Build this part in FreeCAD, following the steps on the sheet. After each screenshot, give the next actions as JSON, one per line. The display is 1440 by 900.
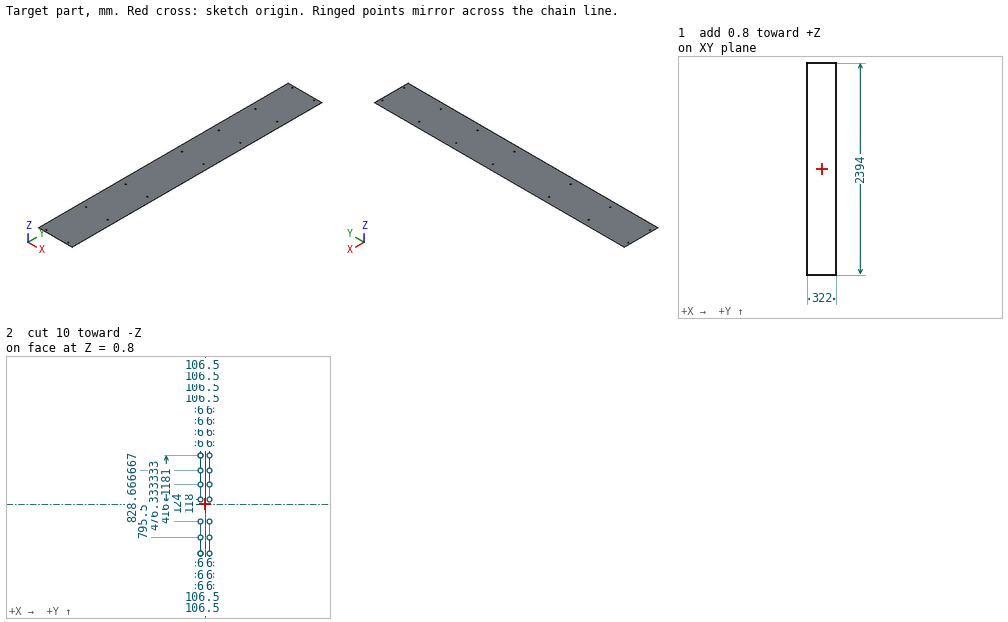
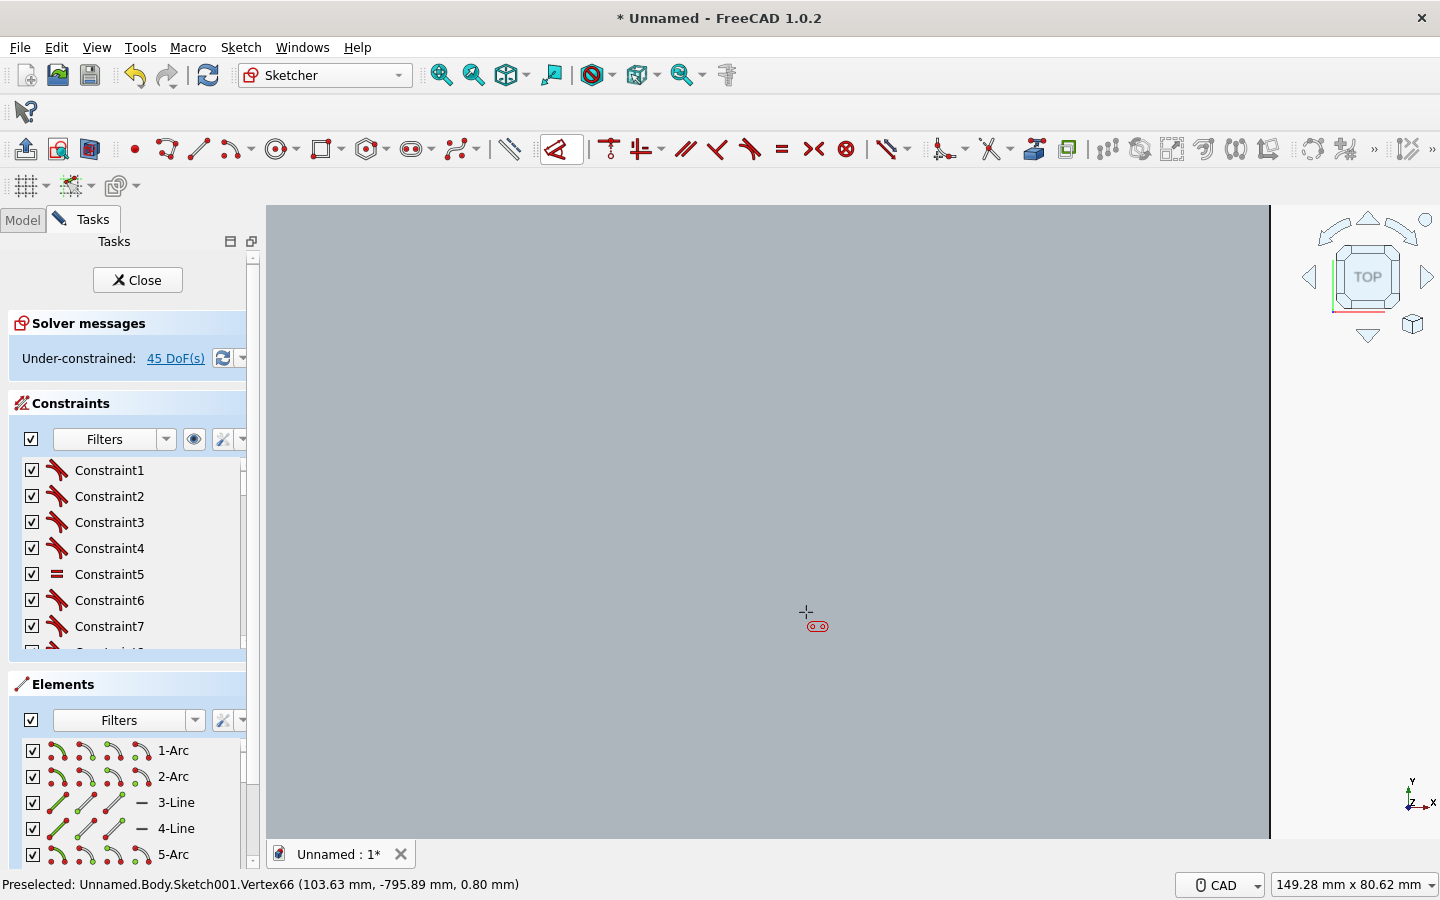
{"action": "scroll", "coordinate": [806, 612], "scroll_direction": "down", "scroll_amount": 18}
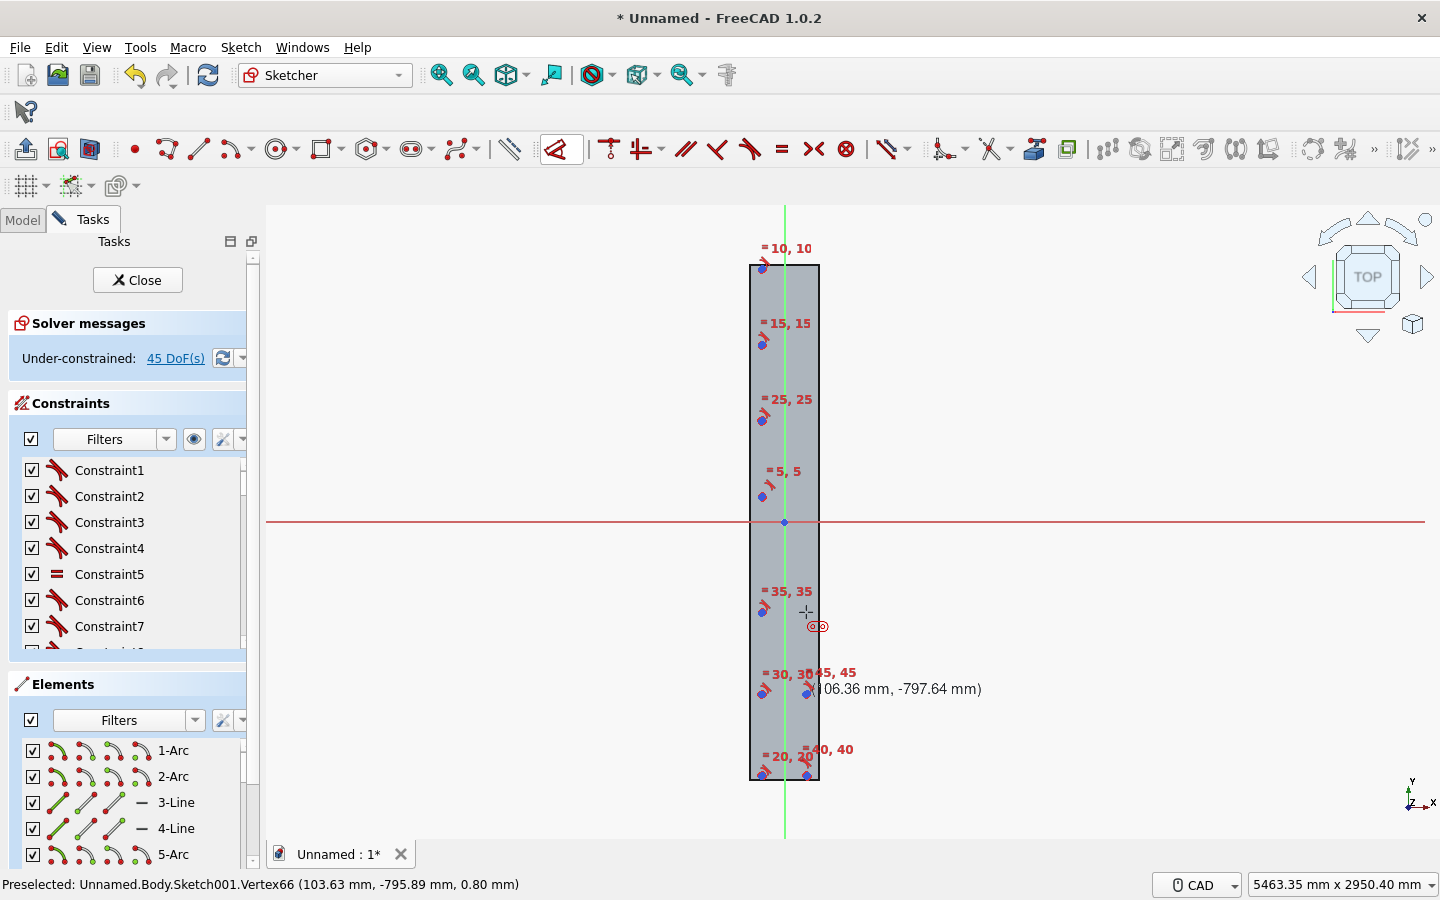
{"action": "left_click", "coordinate": [806, 612]}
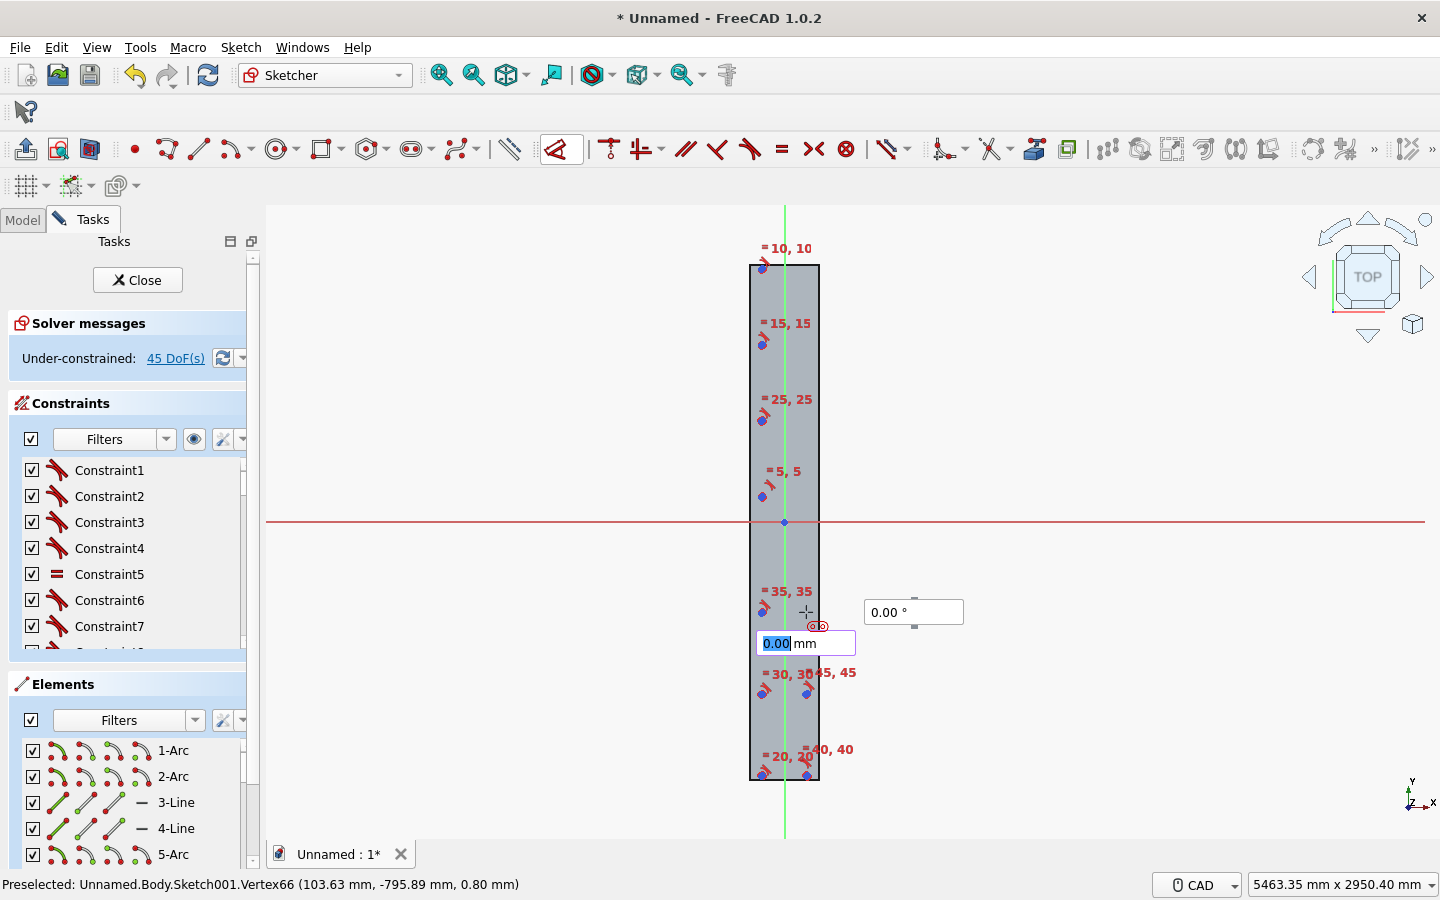
{"action": "scroll", "coordinate": [807, 612], "scroll_direction": "up", "scroll_amount": 13}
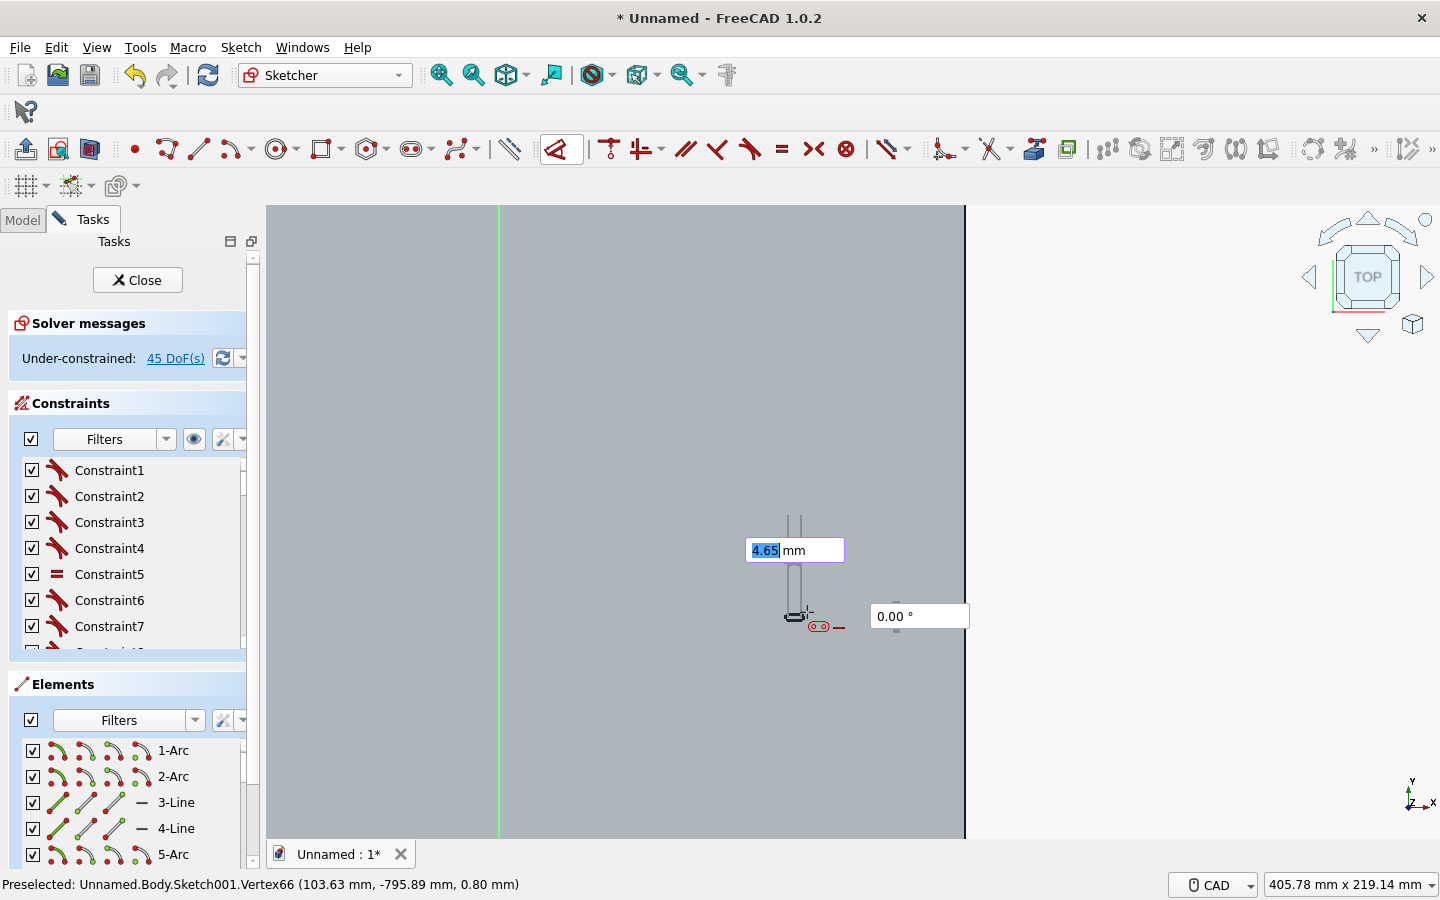
{"action": "left_click", "coordinate": [807, 604]}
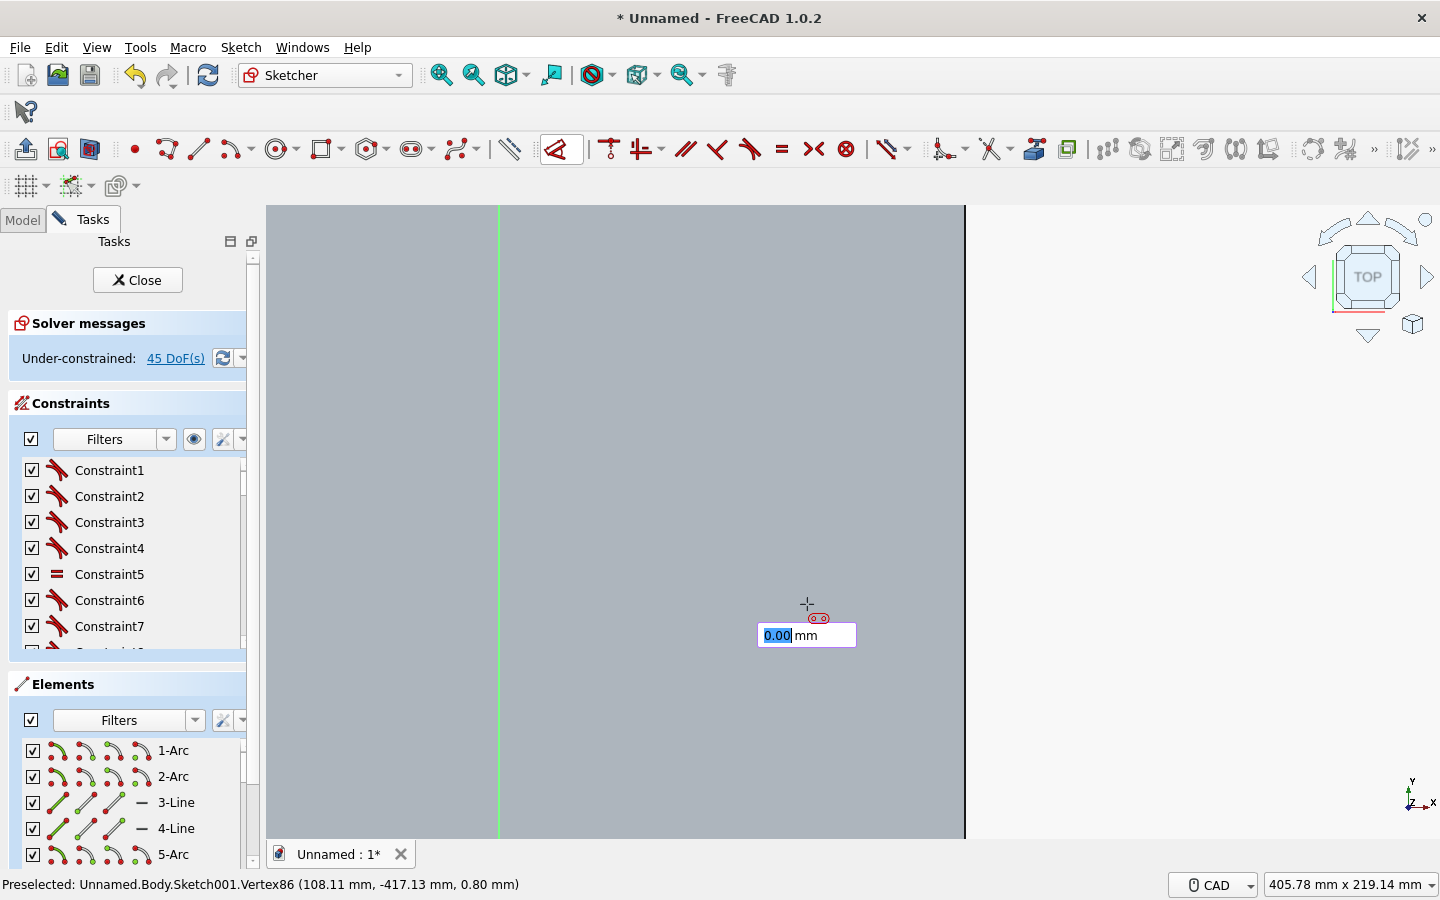
{"action": "scroll", "coordinate": [798, 600], "scroll_direction": "up", "scroll_amount": 4}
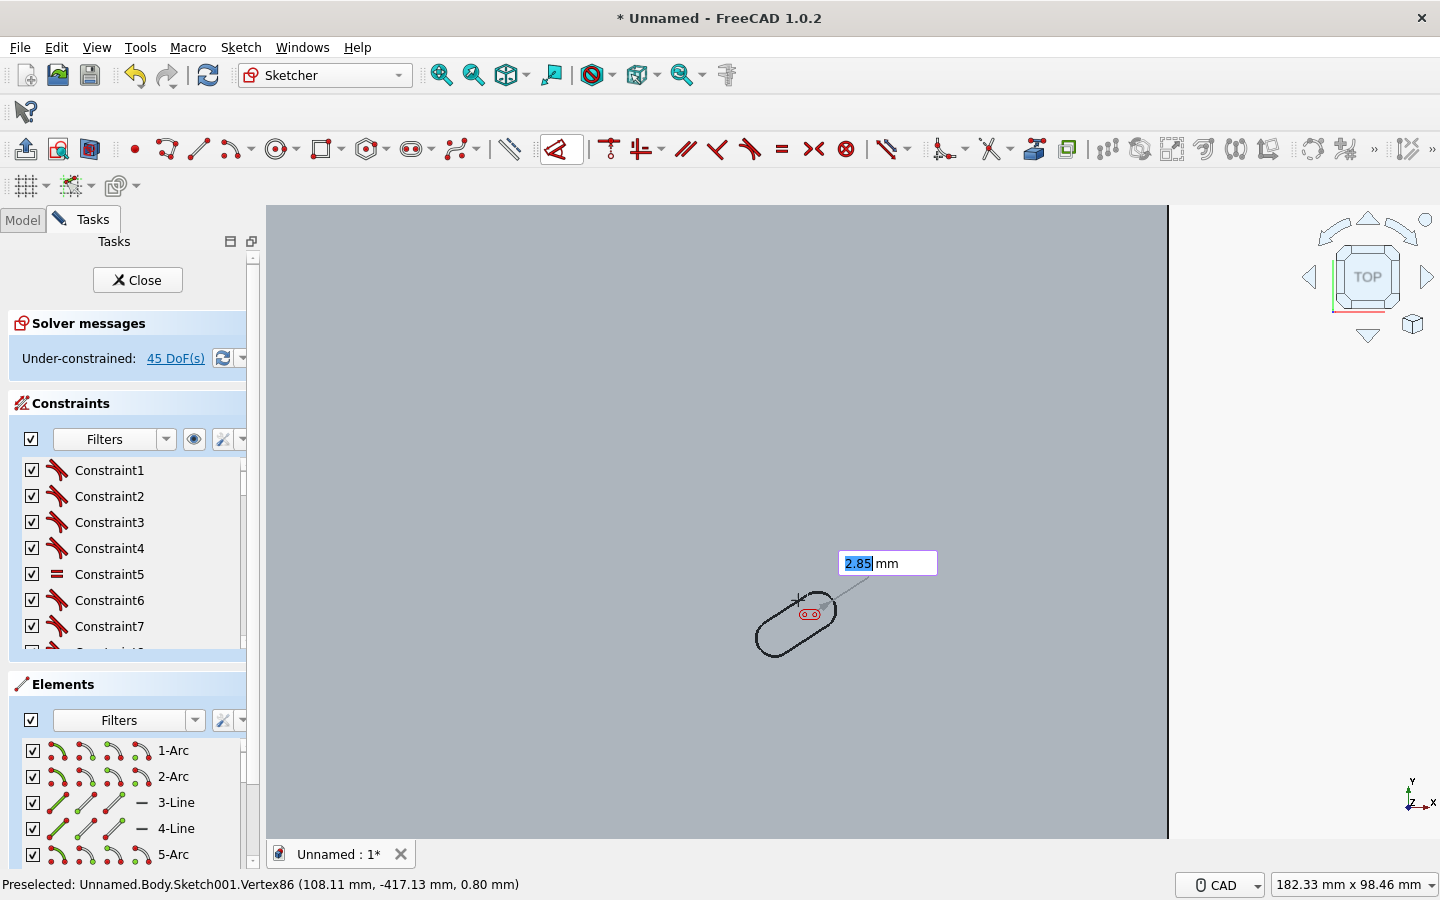
{"action": "left_click", "coordinate": [798, 599]}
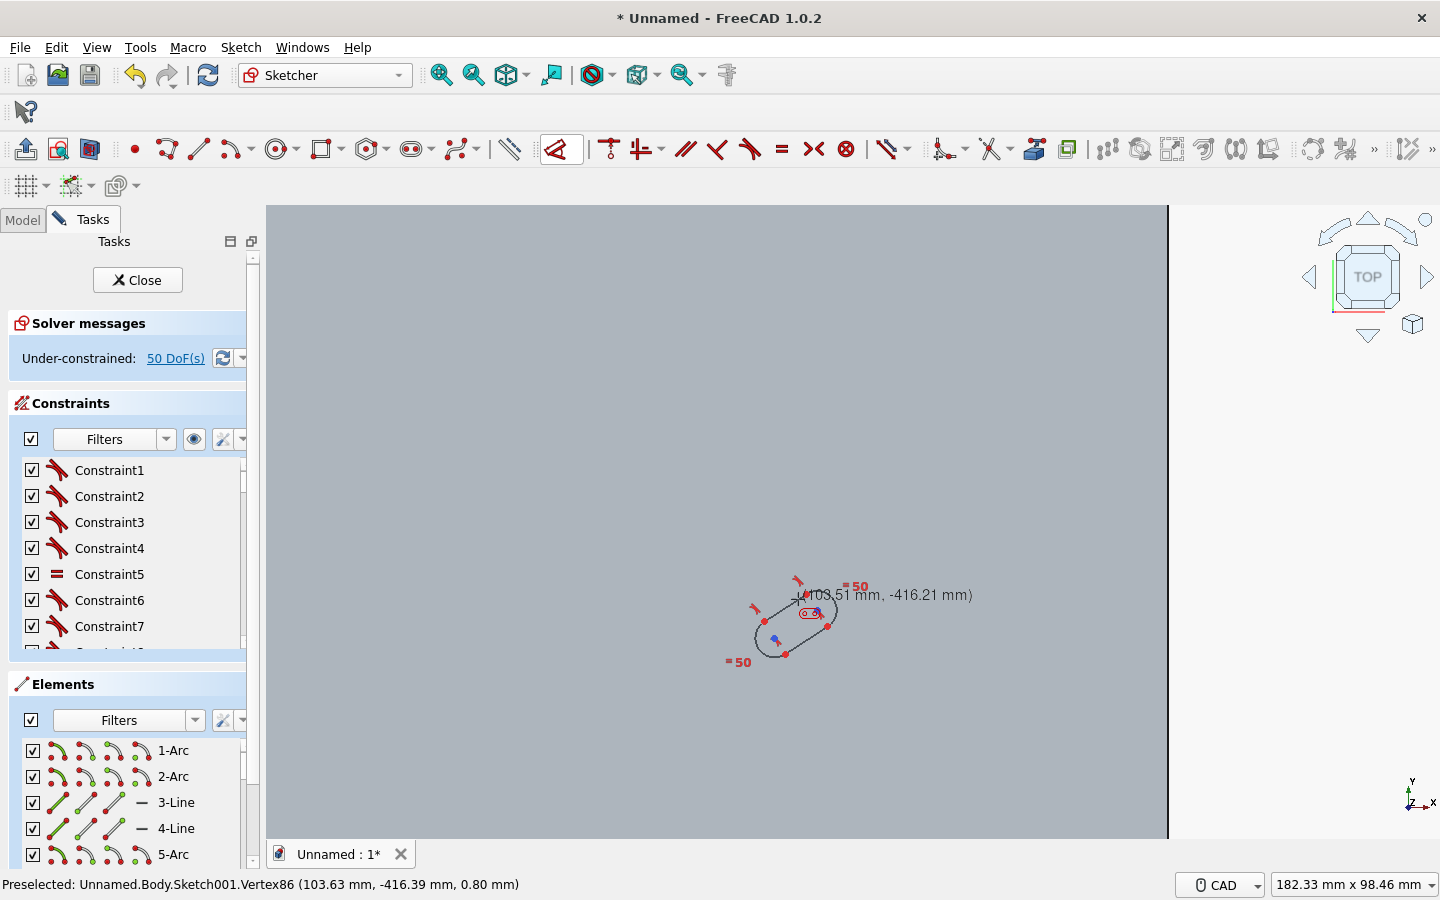
{"action": "scroll", "coordinate": [807, 612], "scroll_direction": "down", "scroll_amount": 17}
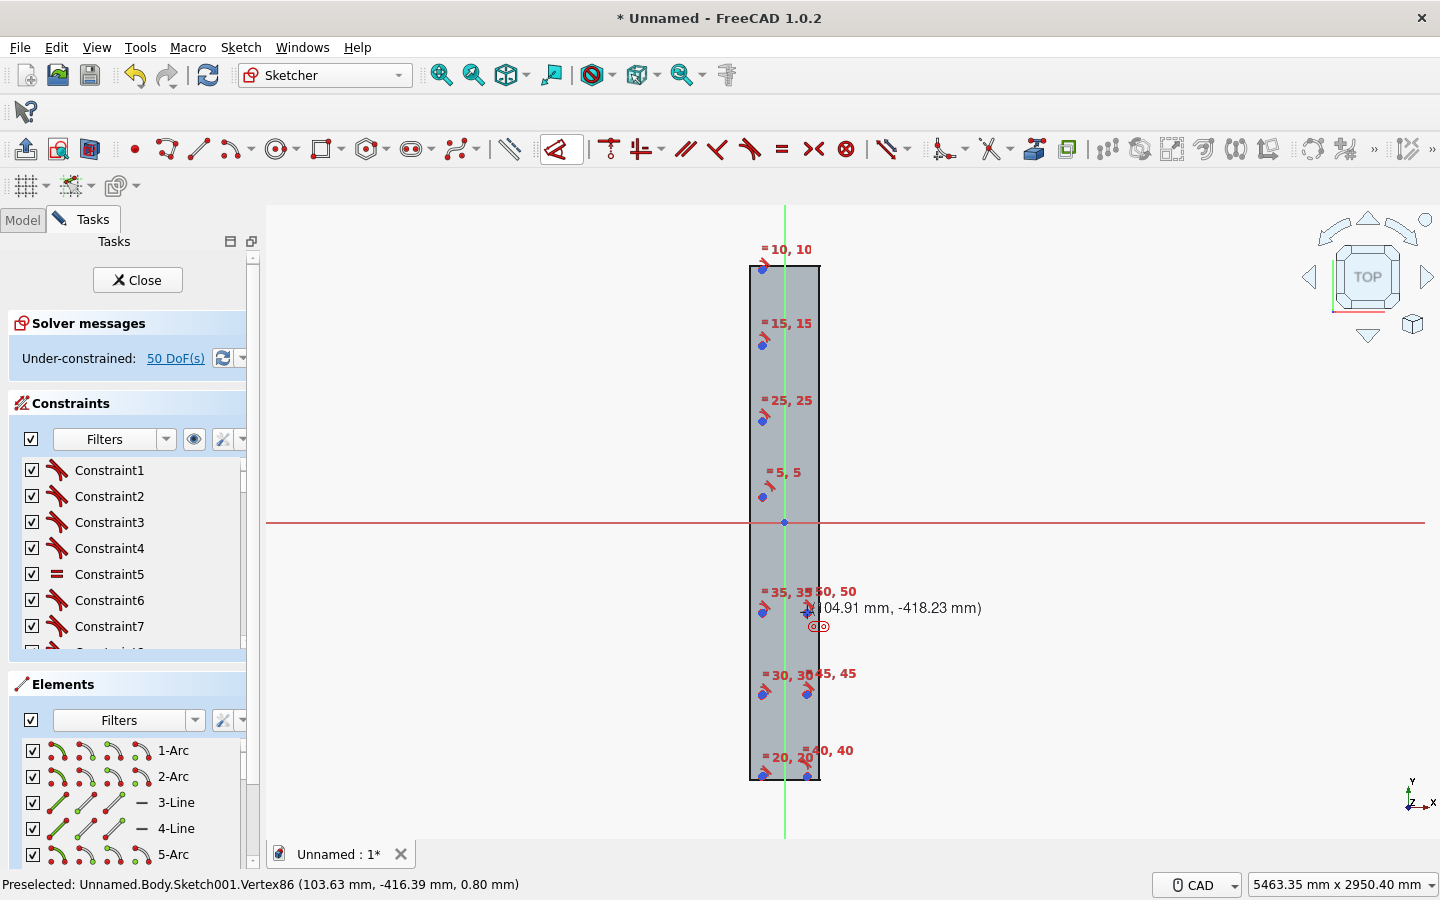
{"action": "scroll", "coordinate": [806, 421], "scroll_direction": "up", "scroll_amount": 18}